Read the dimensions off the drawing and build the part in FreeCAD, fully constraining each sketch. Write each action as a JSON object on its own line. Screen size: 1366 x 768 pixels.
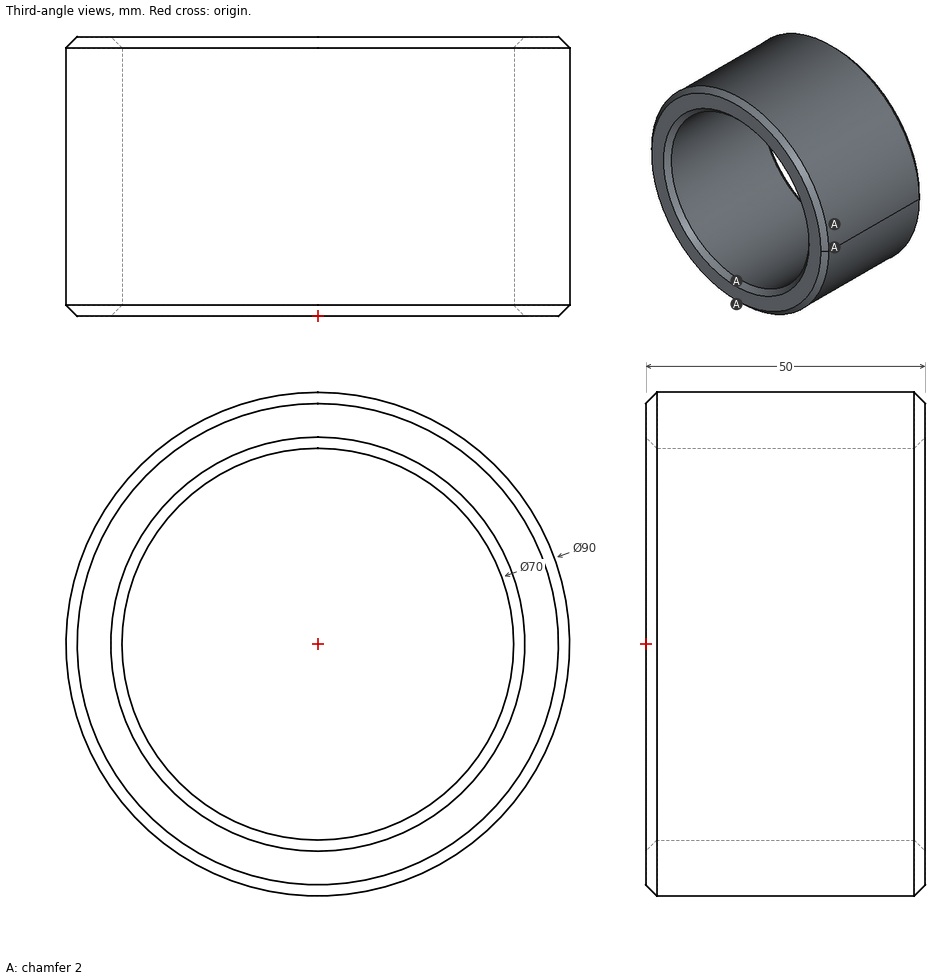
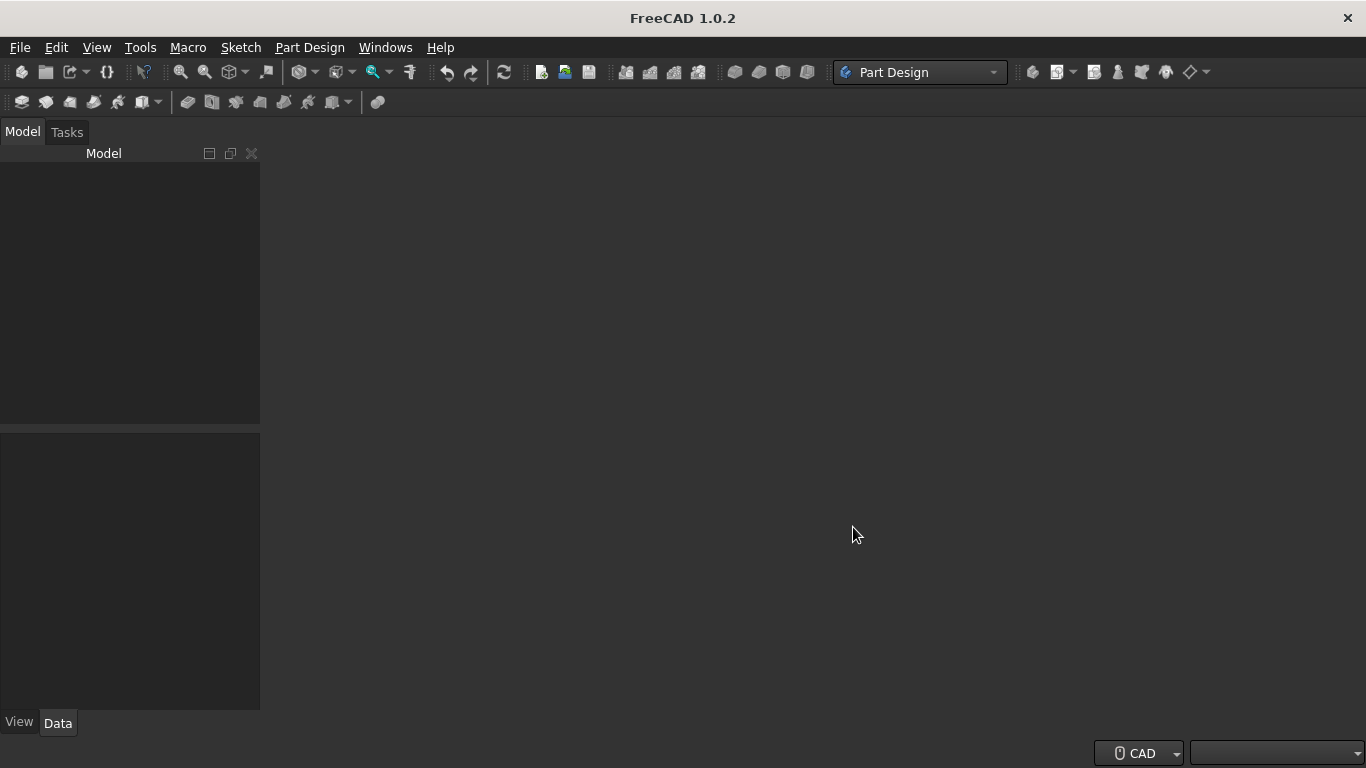
{"action": "left_click", "coordinate": [542, 72]}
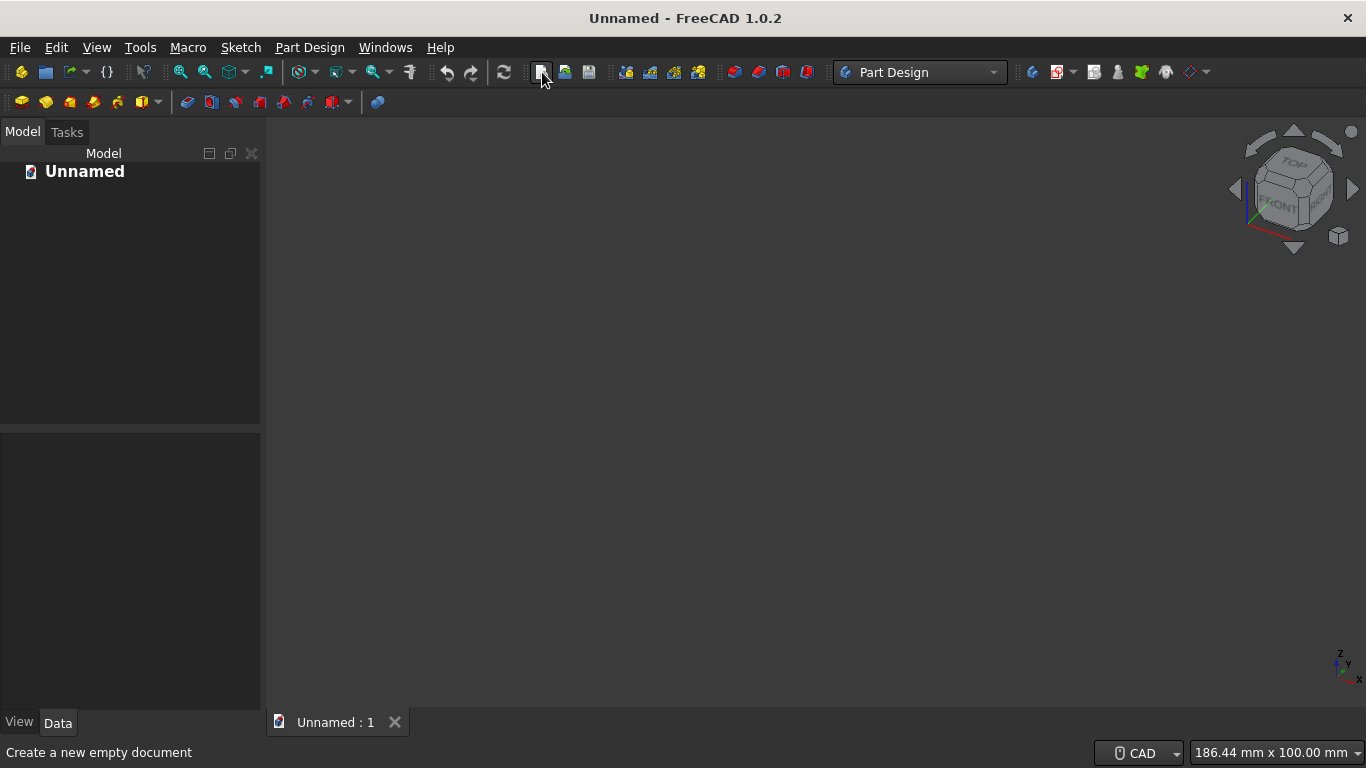
{"action": "left_click", "coordinate": [1058, 72]}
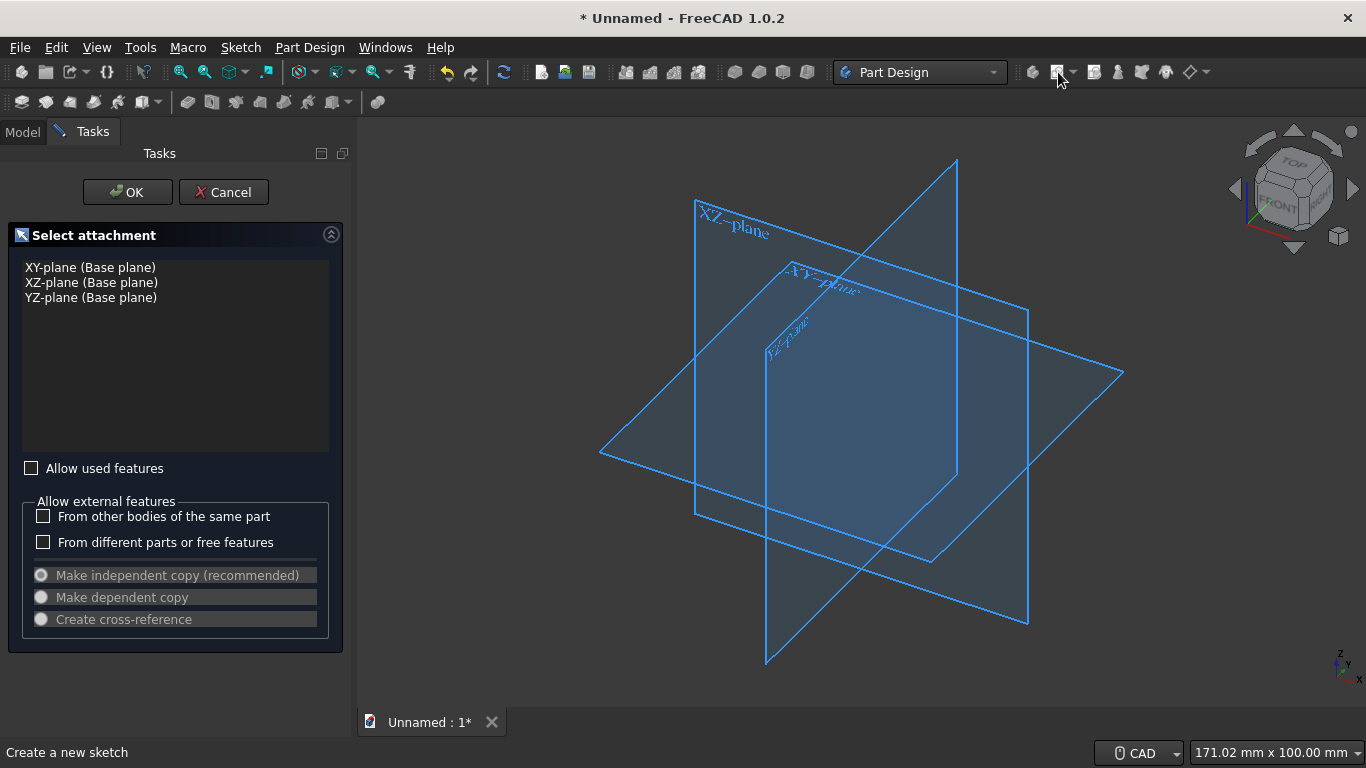
{"action": "left_click", "coordinate": [82, 282]}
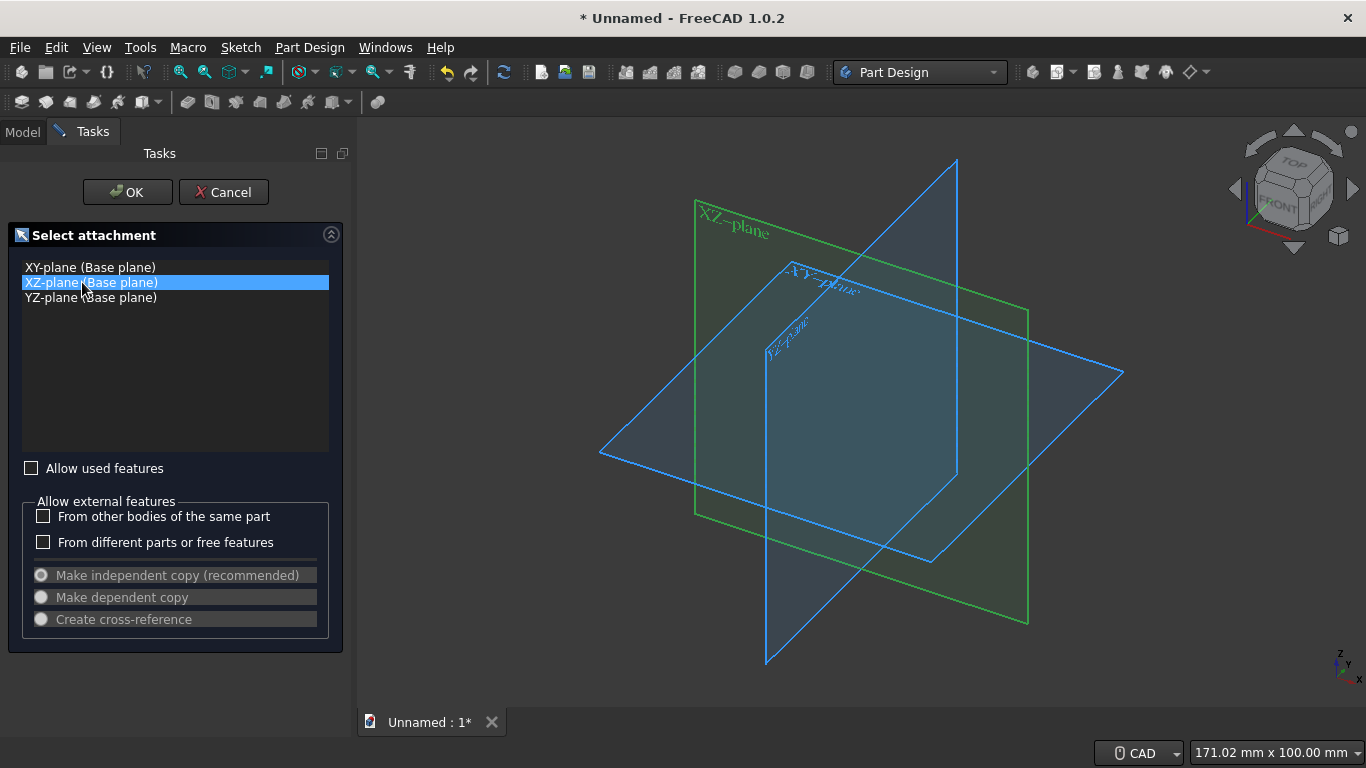
{"action": "left_click", "coordinate": [128, 192]}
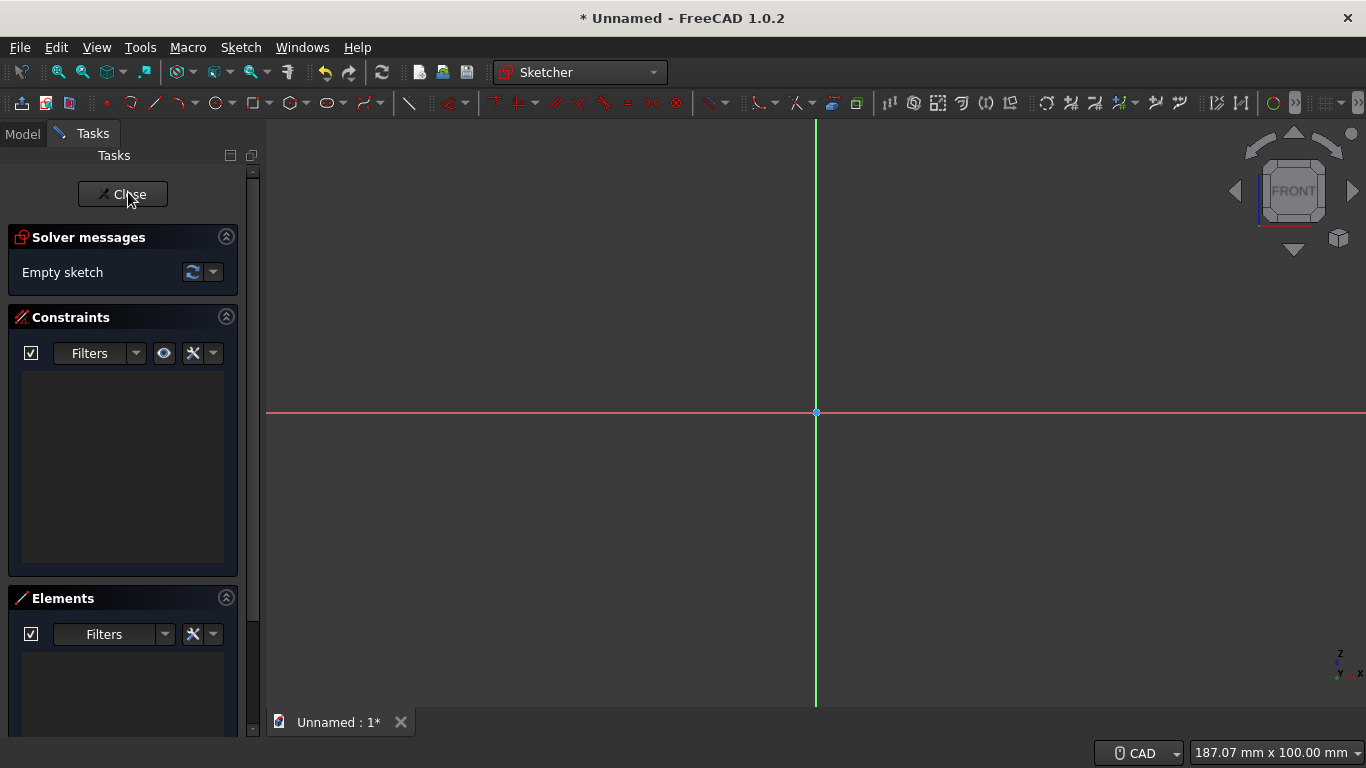
{"action": "scroll", "coordinate": [608, 413], "scroll_direction": "down", "scroll_amount": 2}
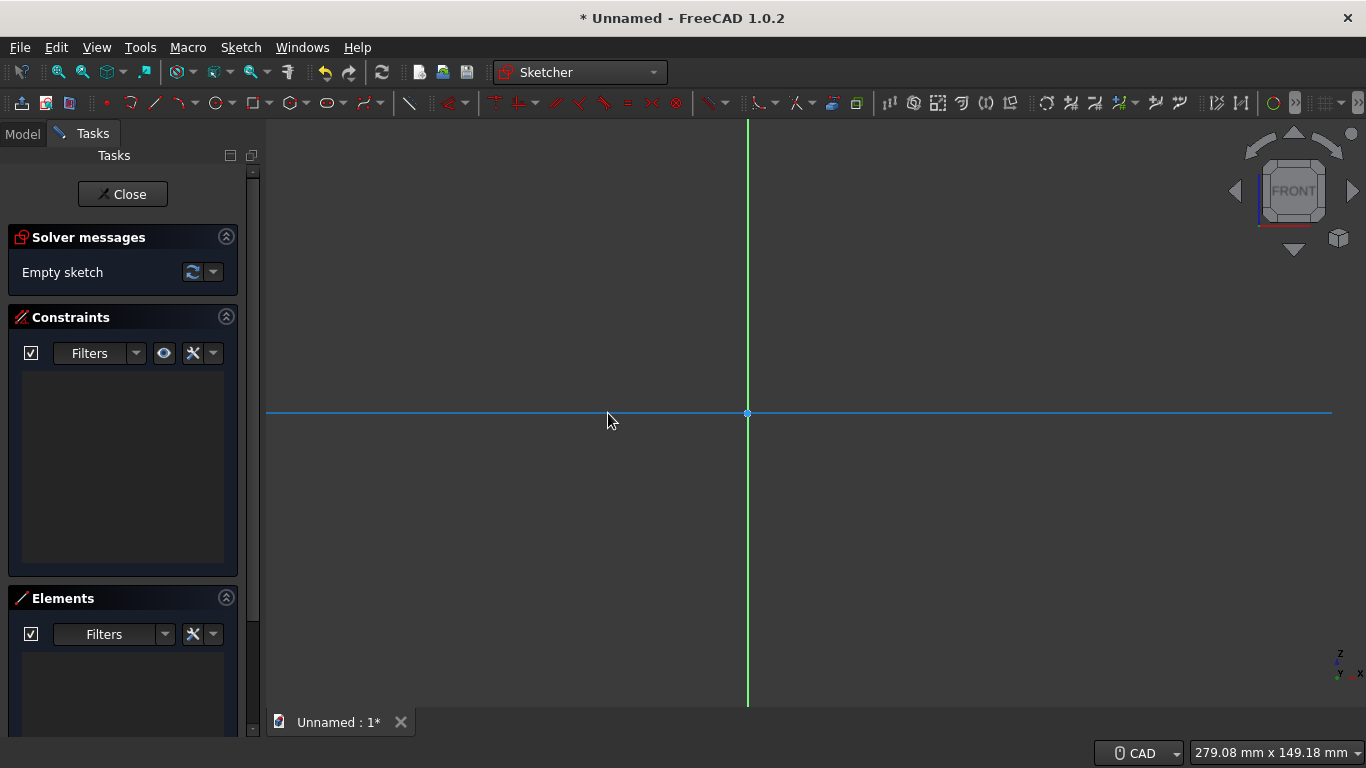
{"action": "left_click", "coordinate": [216, 104]}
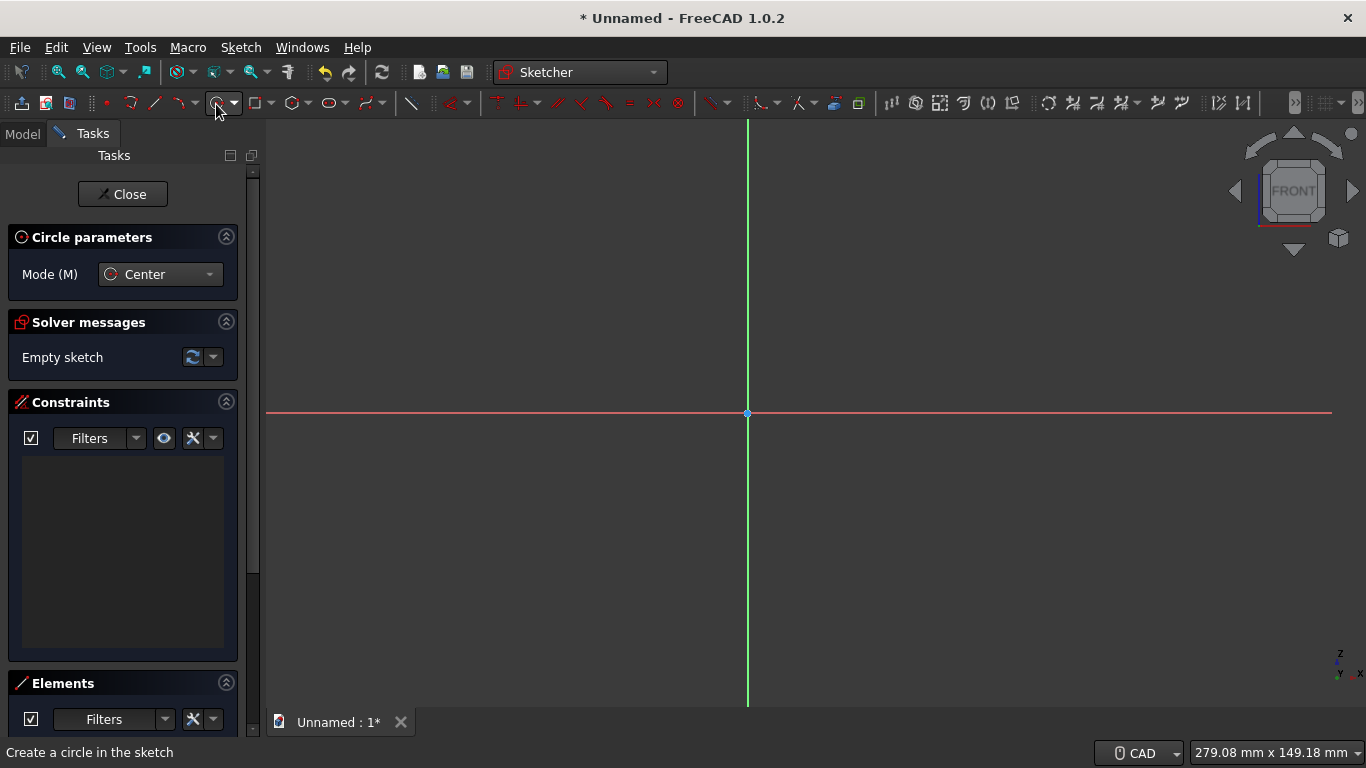
{"action": "left_click", "coordinate": [748, 413]}
{"action": "left_click", "coordinate": [873, 288]}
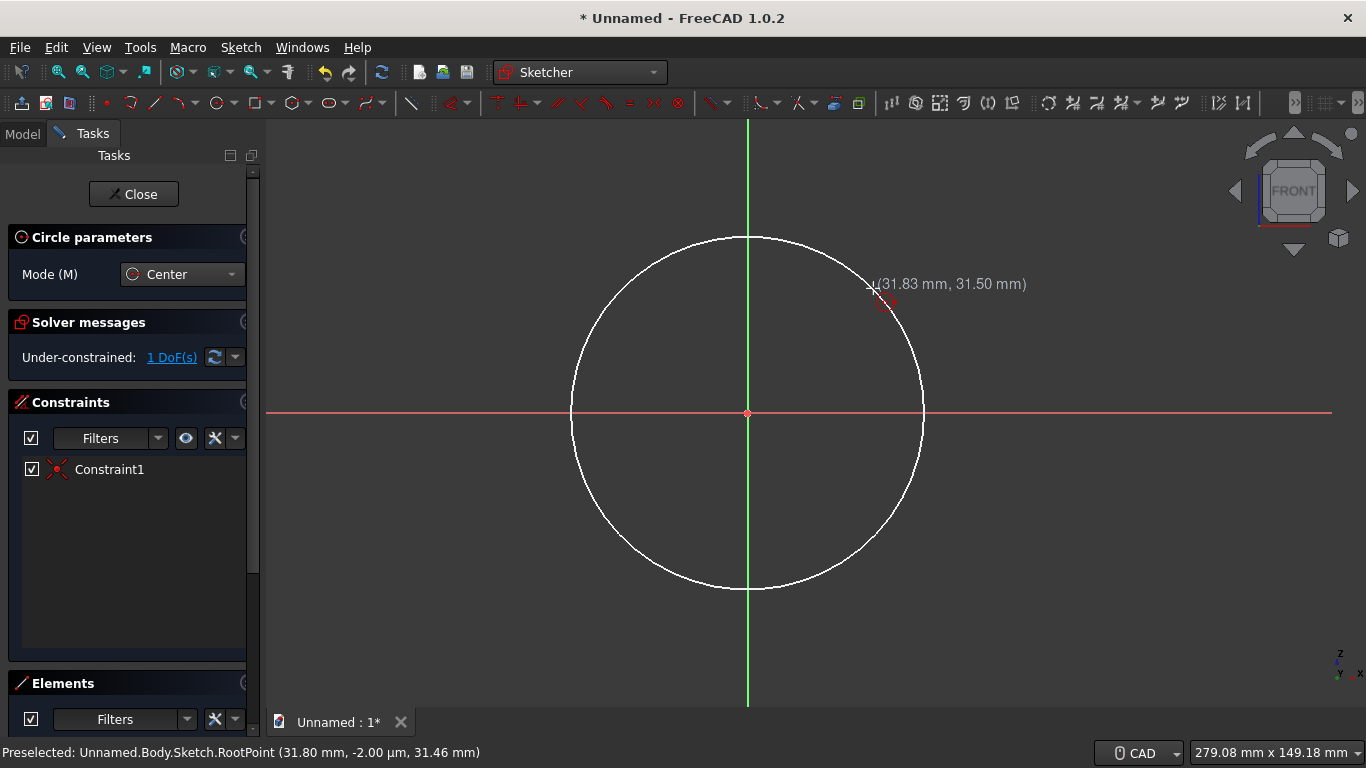
{"action": "left_click", "coordinate": [748, 413]}
{"action": "left_click", "coordinate": [845, 316]}
{"action": "key", "text": "Escape"}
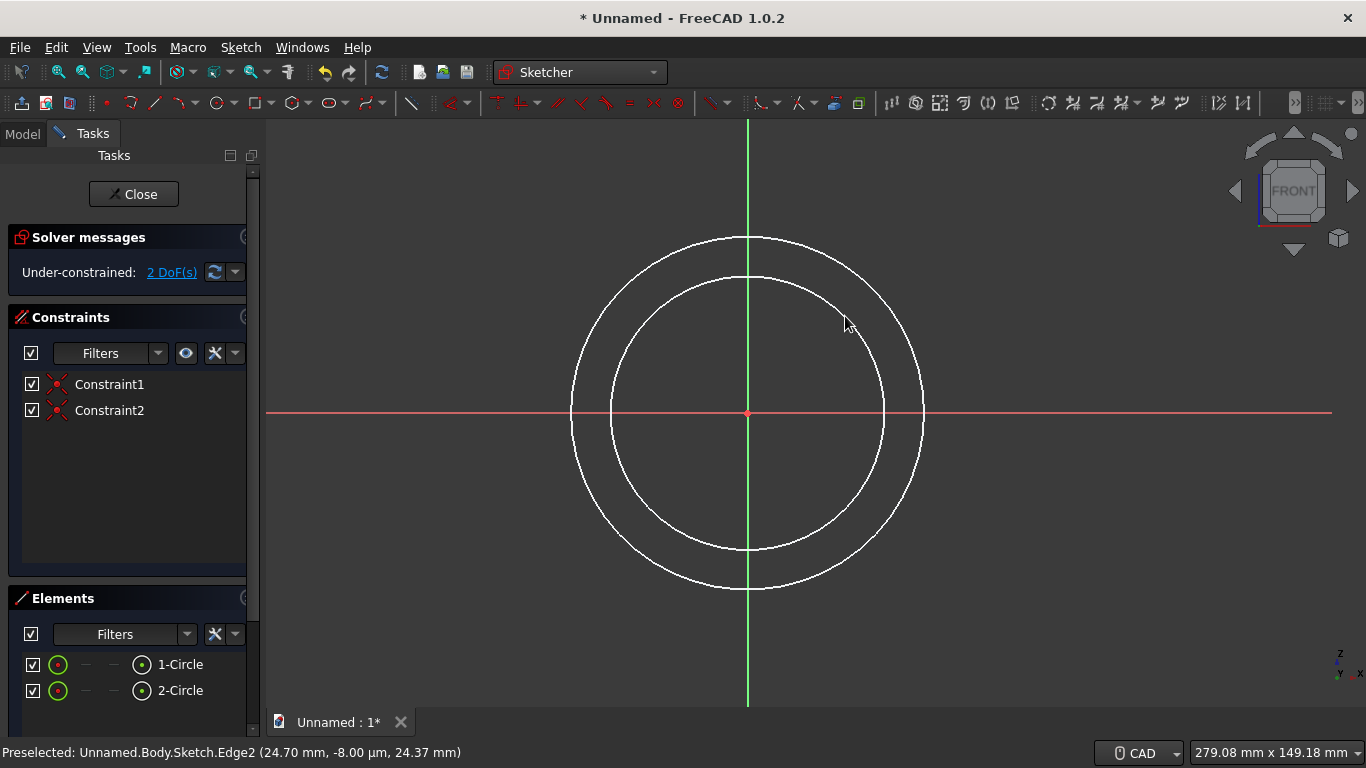
{"action": "left_click", "coordinate": [450, 104]}